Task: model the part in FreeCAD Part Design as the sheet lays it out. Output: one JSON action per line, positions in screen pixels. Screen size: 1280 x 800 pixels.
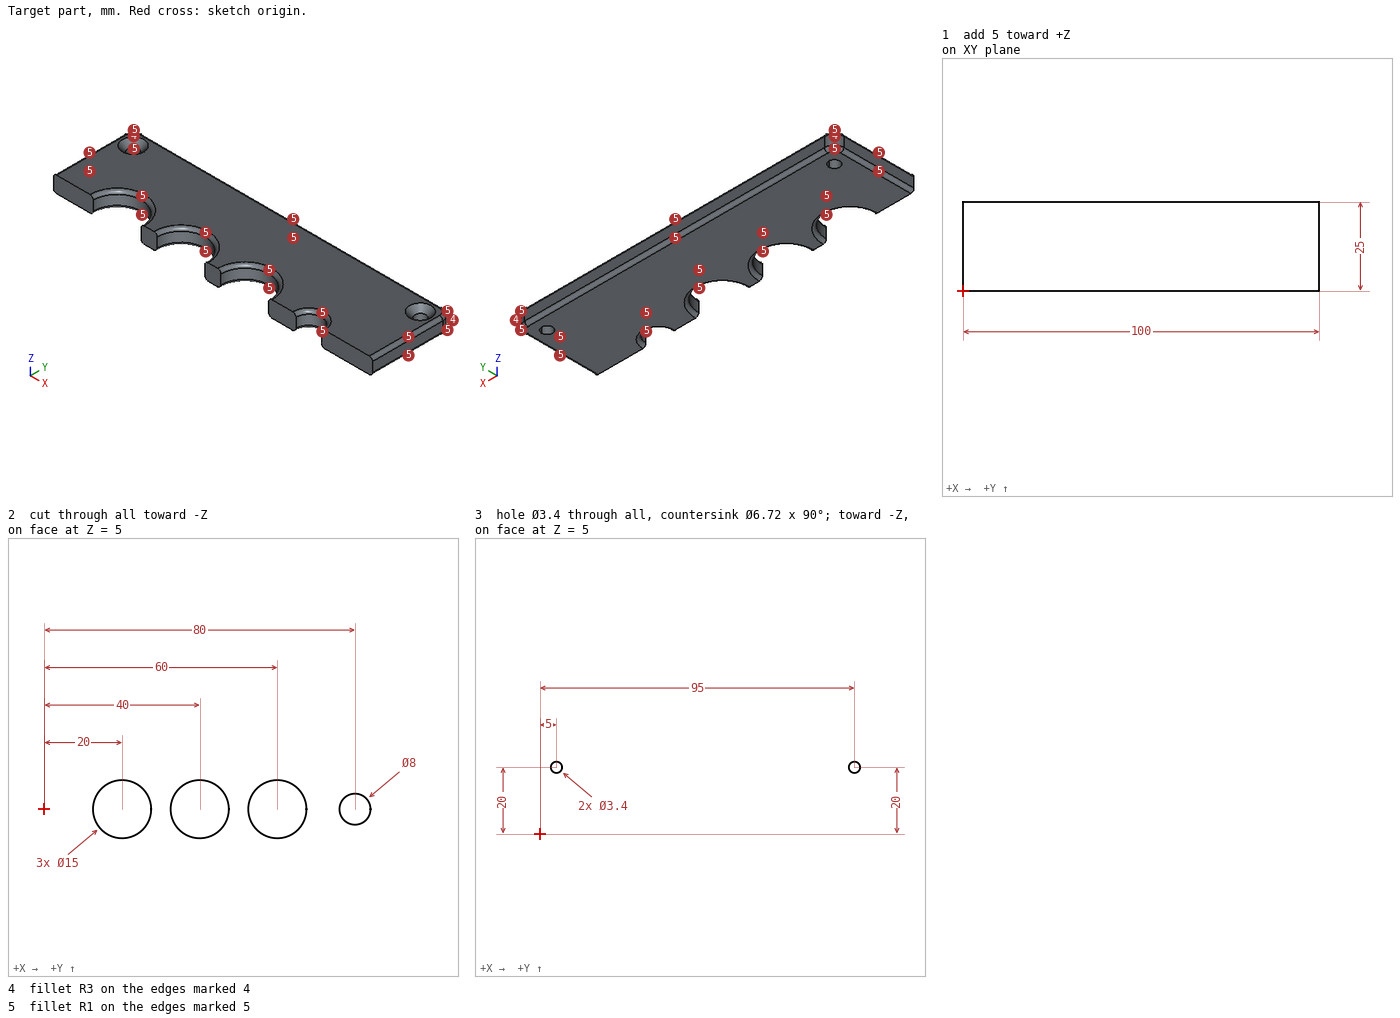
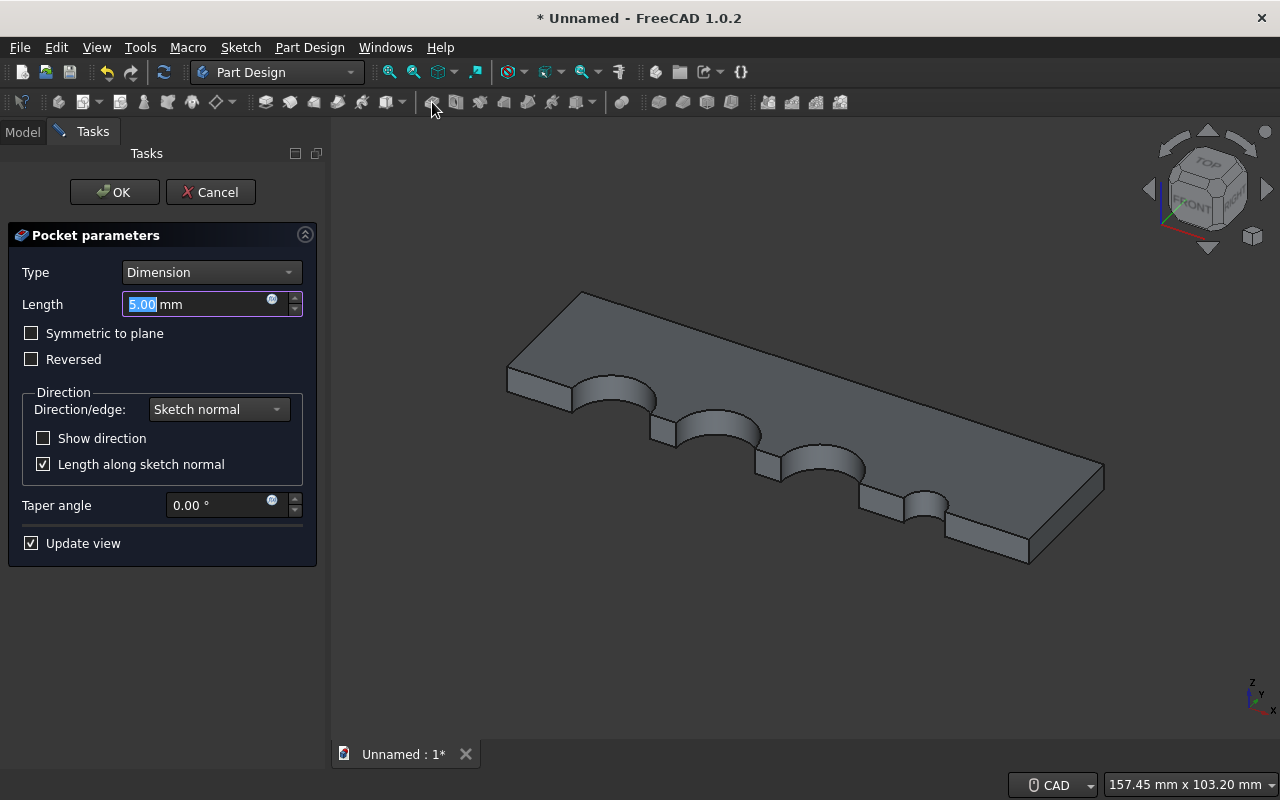
{"action": "left_click", "coordinate": [212, 272]}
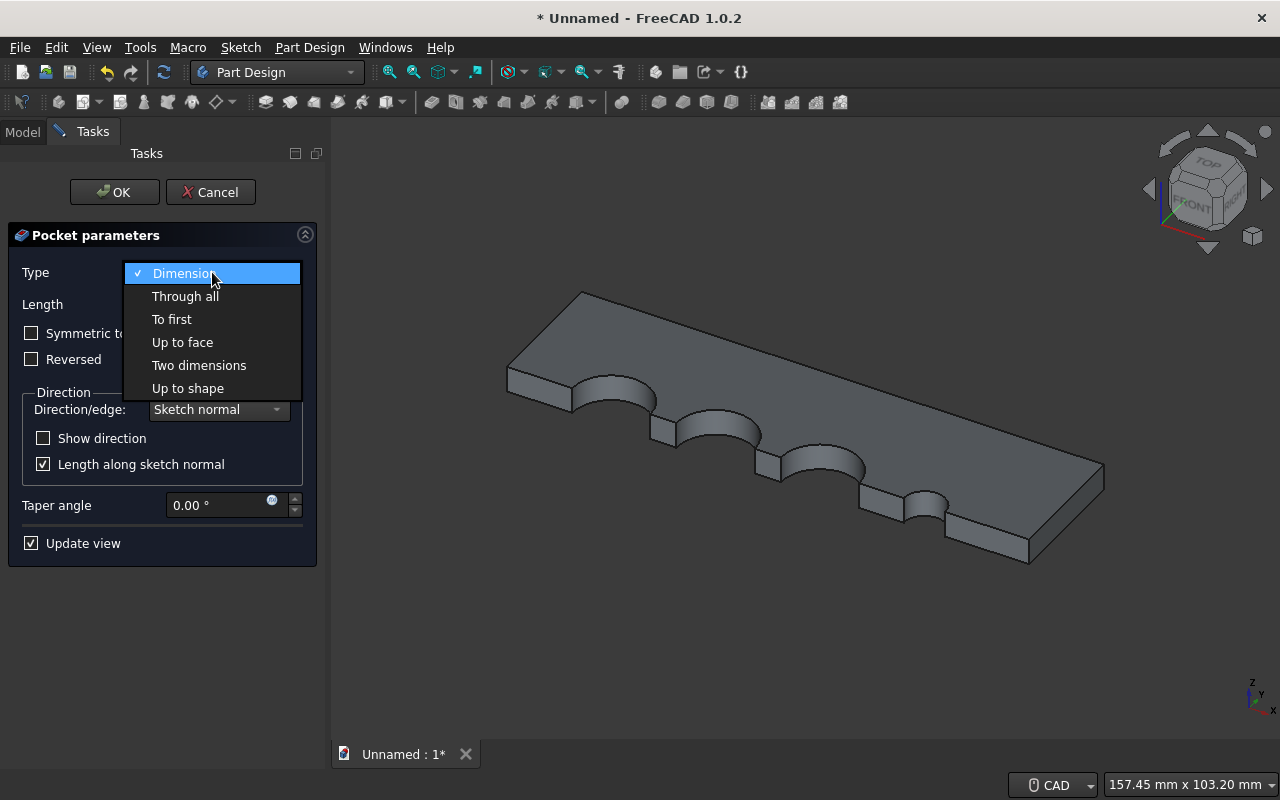
{"action": "left_click", "coordinate": [212, 296]}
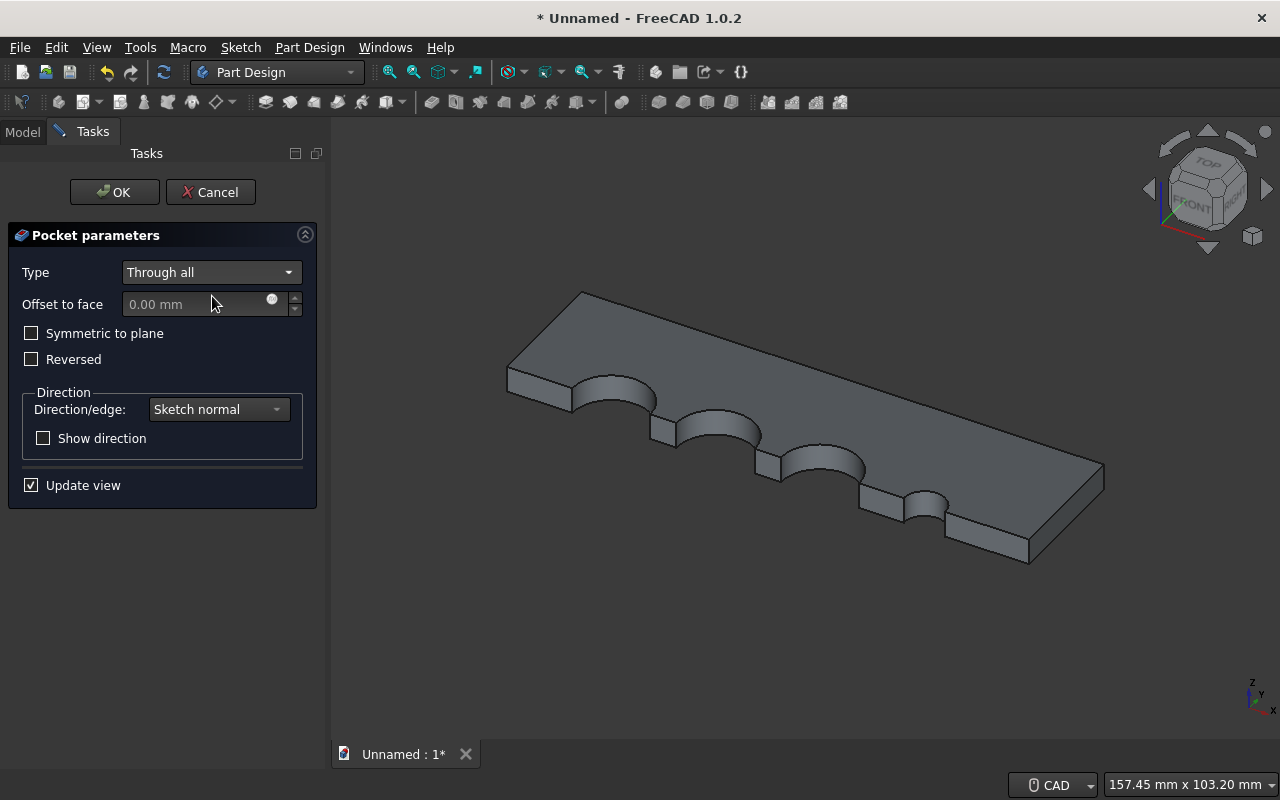
{"action": "left_click", "coordinate": [115, 192]}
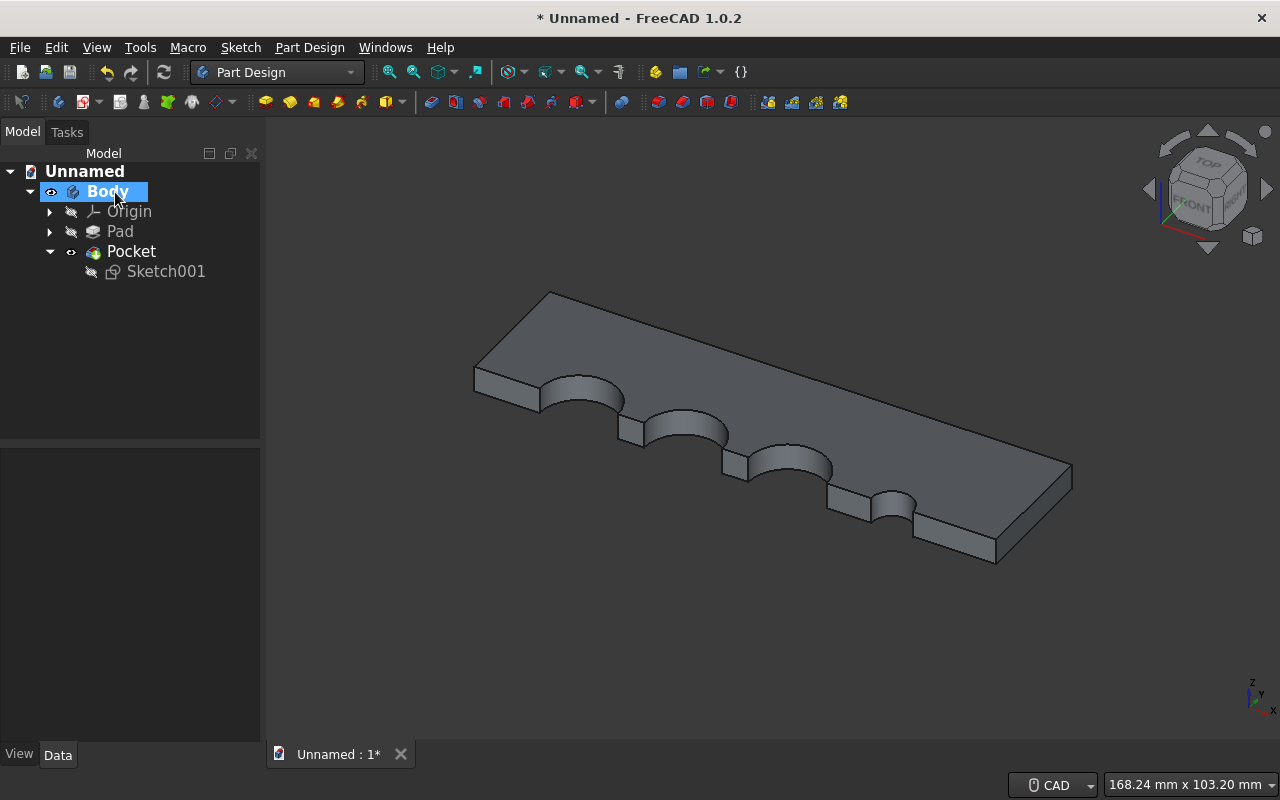
{"action": "left_click", "coordinate": [933, 453]}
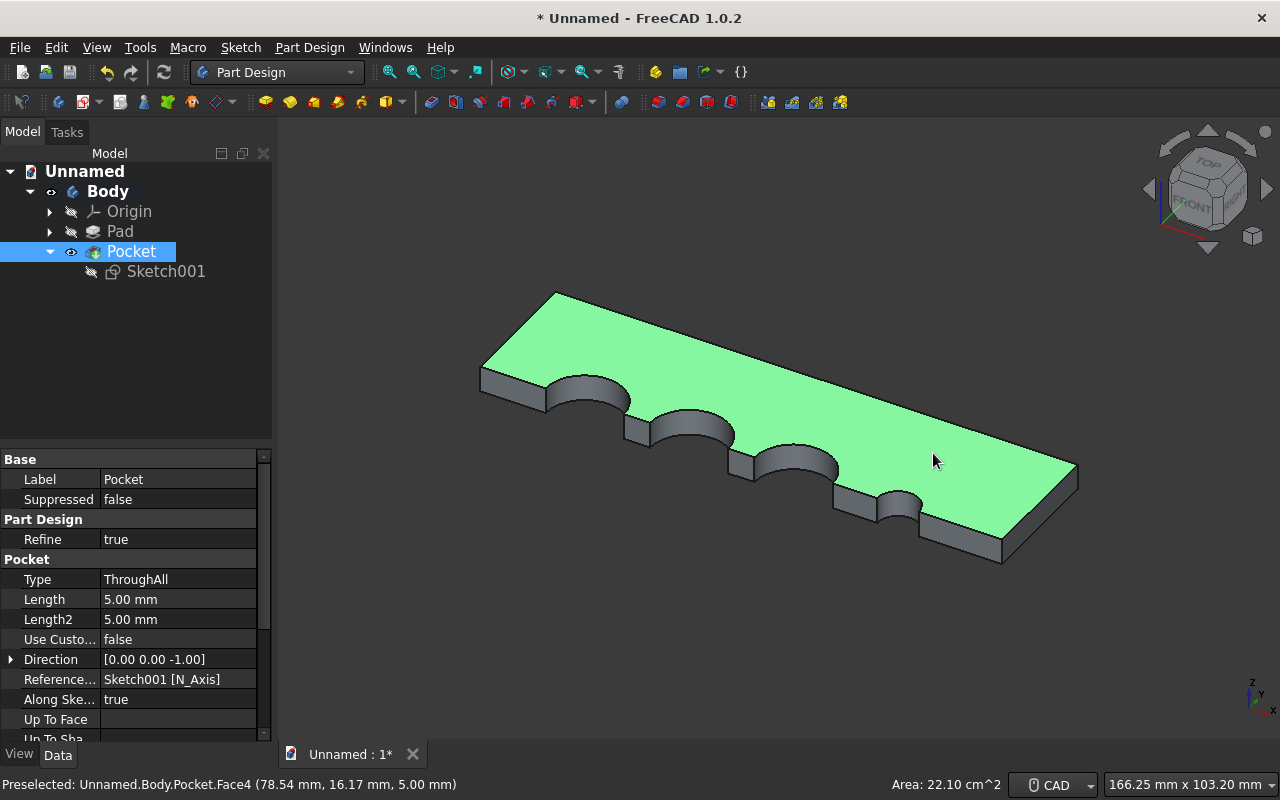
{"action": "left_click", "coordinate": [84, 102]}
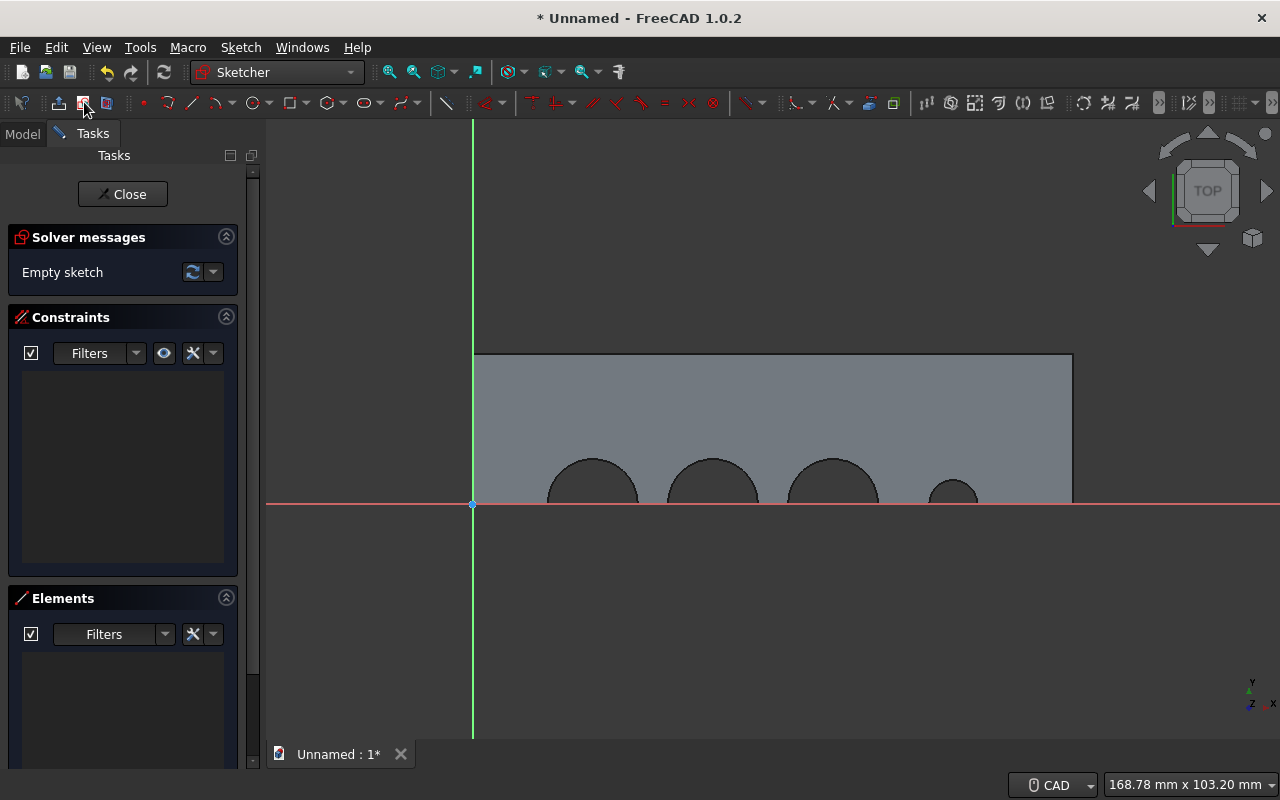
{"action": "key", "text": "g c"}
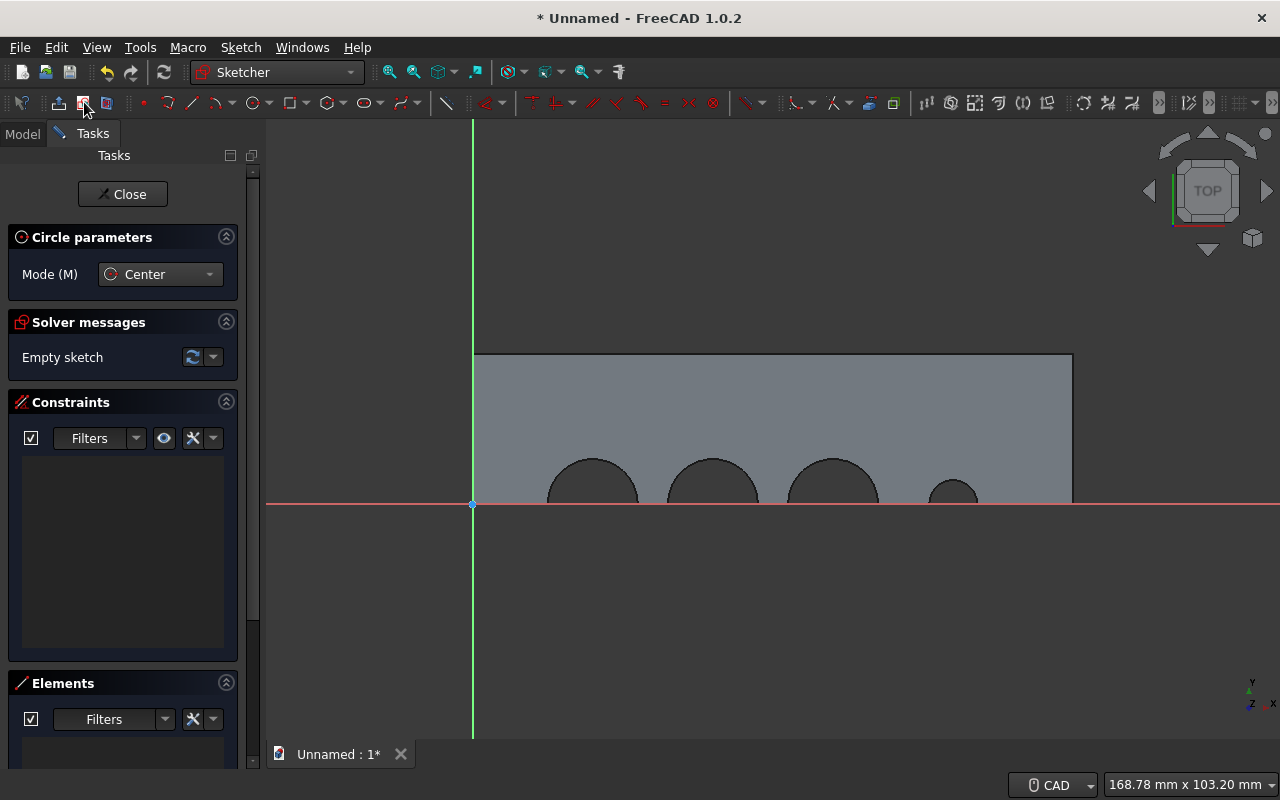
{"action": "scroll", "coordinate": [503, 384], "scroll_direction": "up", "scroll_amount": 4}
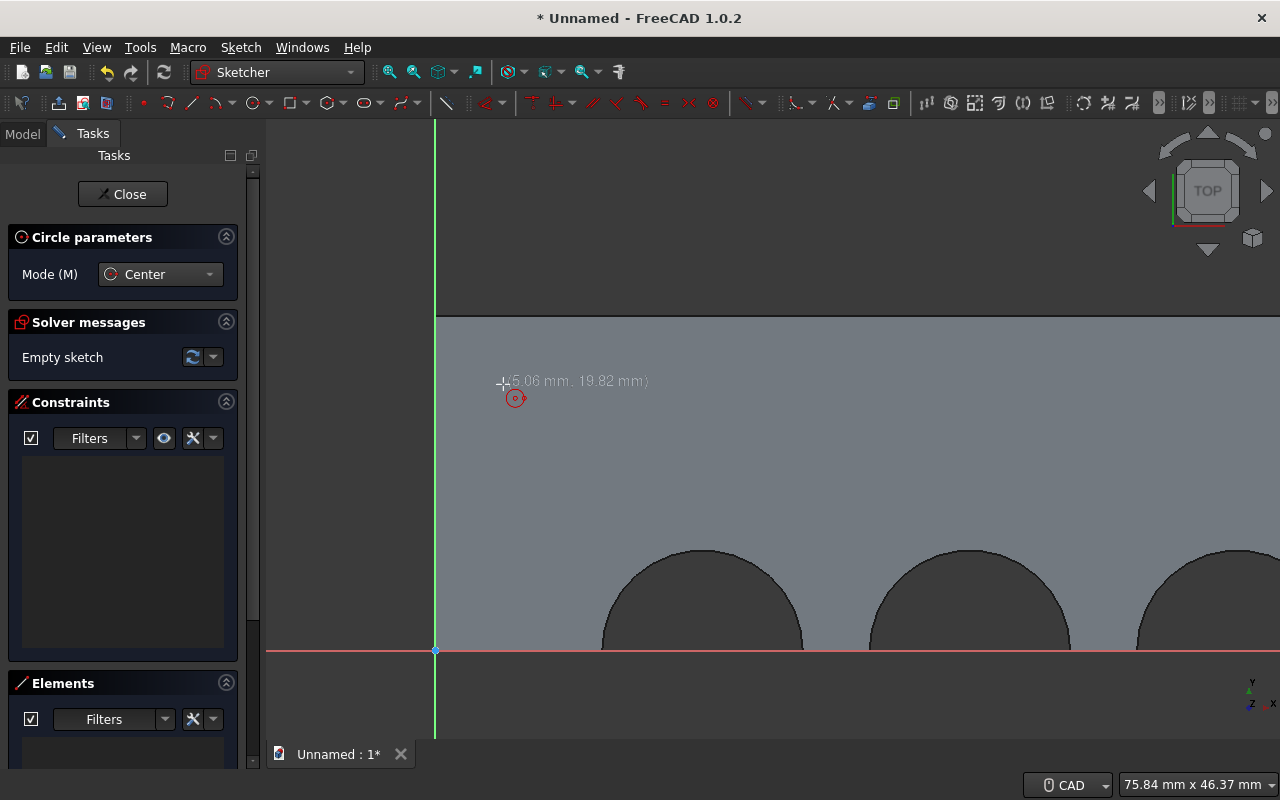
{"action": "left_click", "coordinate": [502, 383]}
{"action": "mouse_move", "coordinate": [518, 367]}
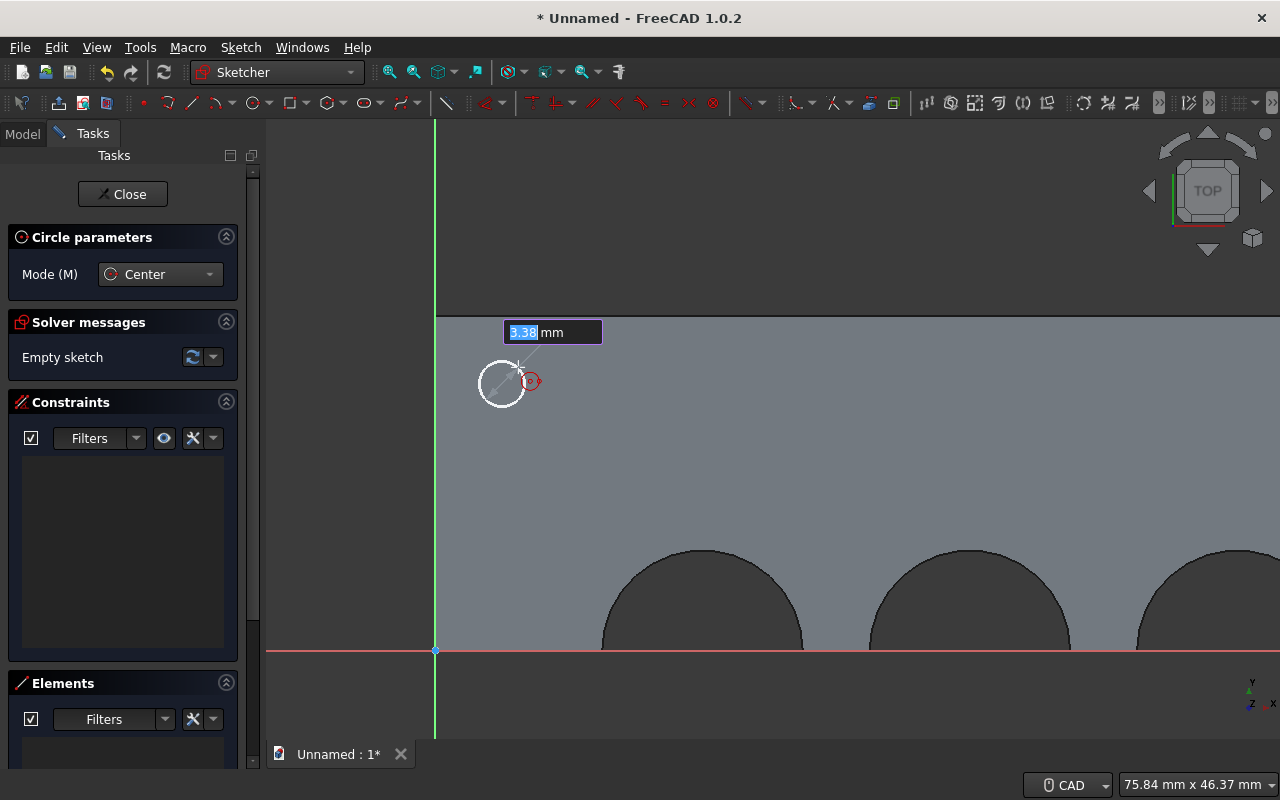
{"action": "type", "text": "3.4"}
{"action": "key", "text": "Return"}